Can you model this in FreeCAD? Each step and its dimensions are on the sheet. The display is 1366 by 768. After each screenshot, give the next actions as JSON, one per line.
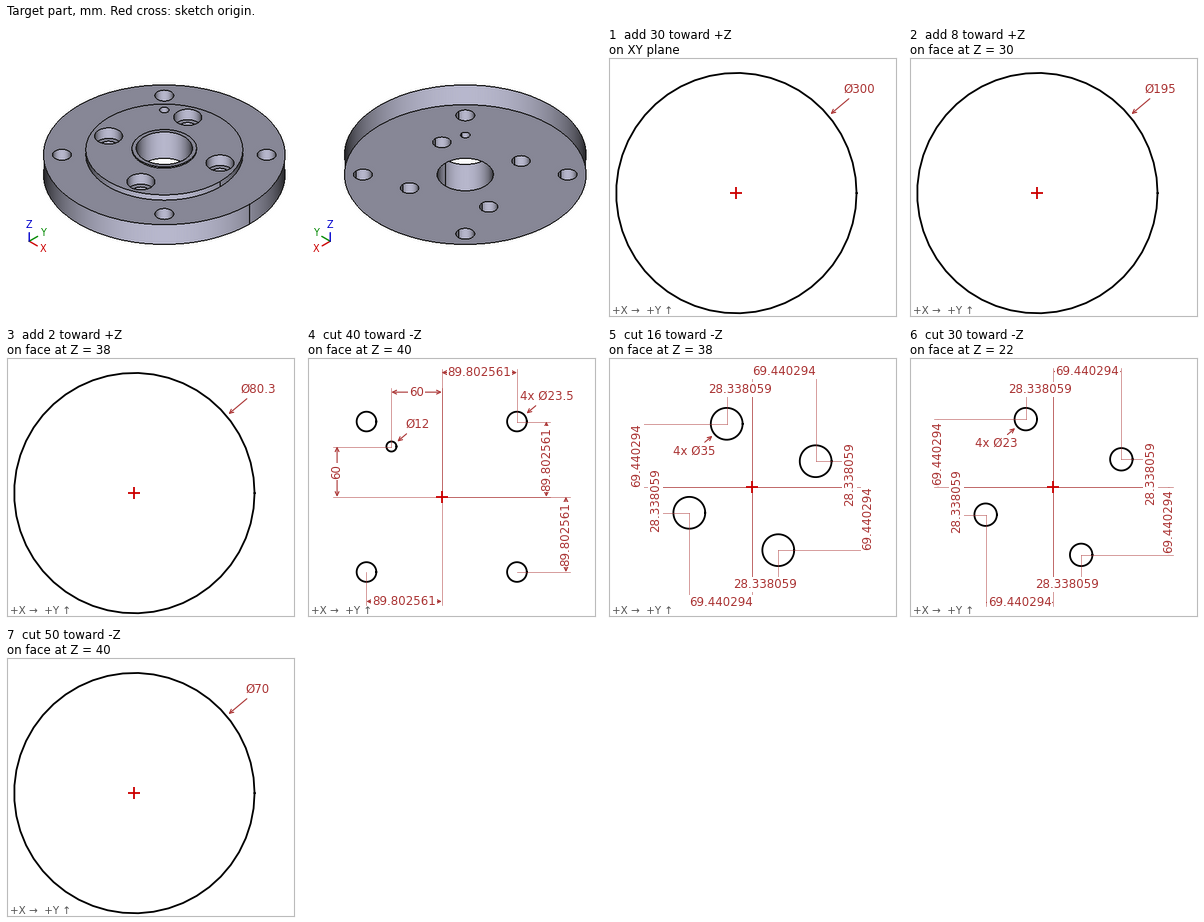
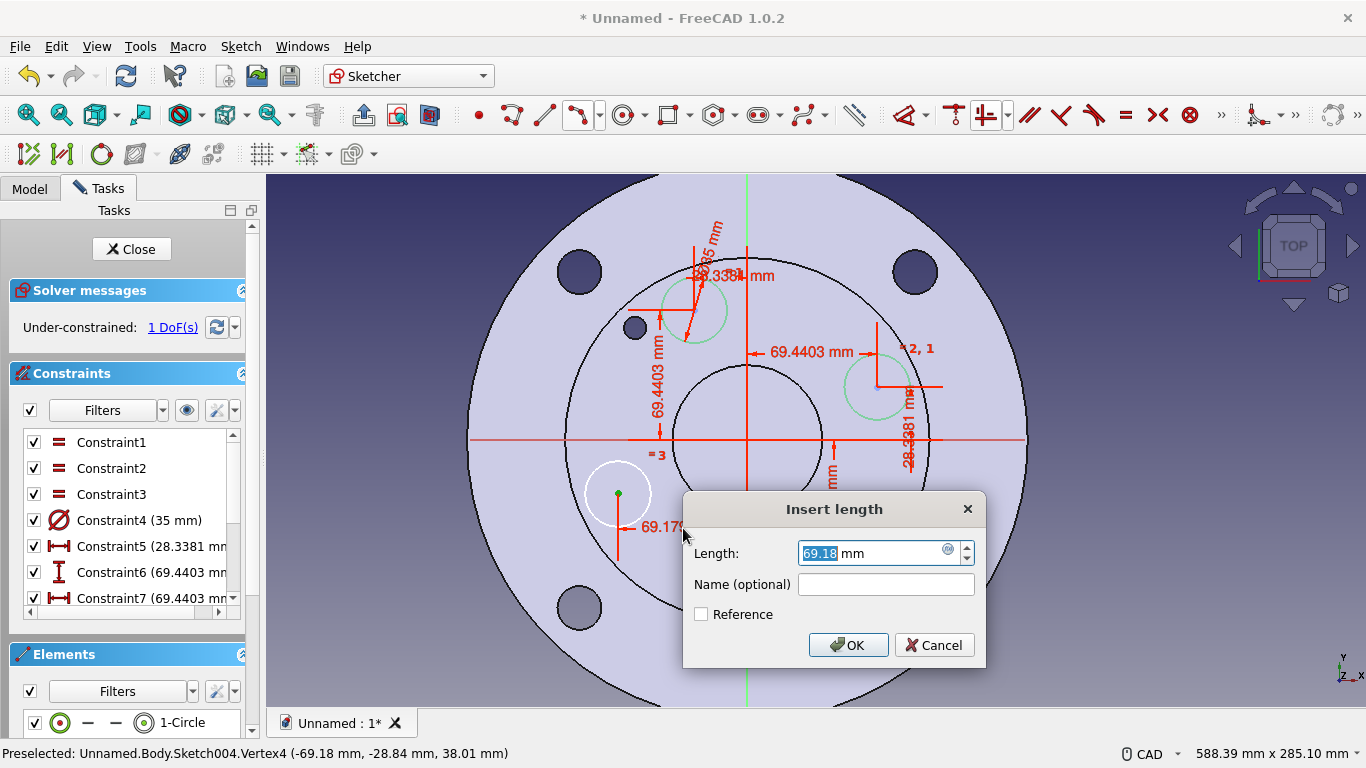
{"action": "type", "text": "69.440294"}
{"action": "key", "text": "Return"}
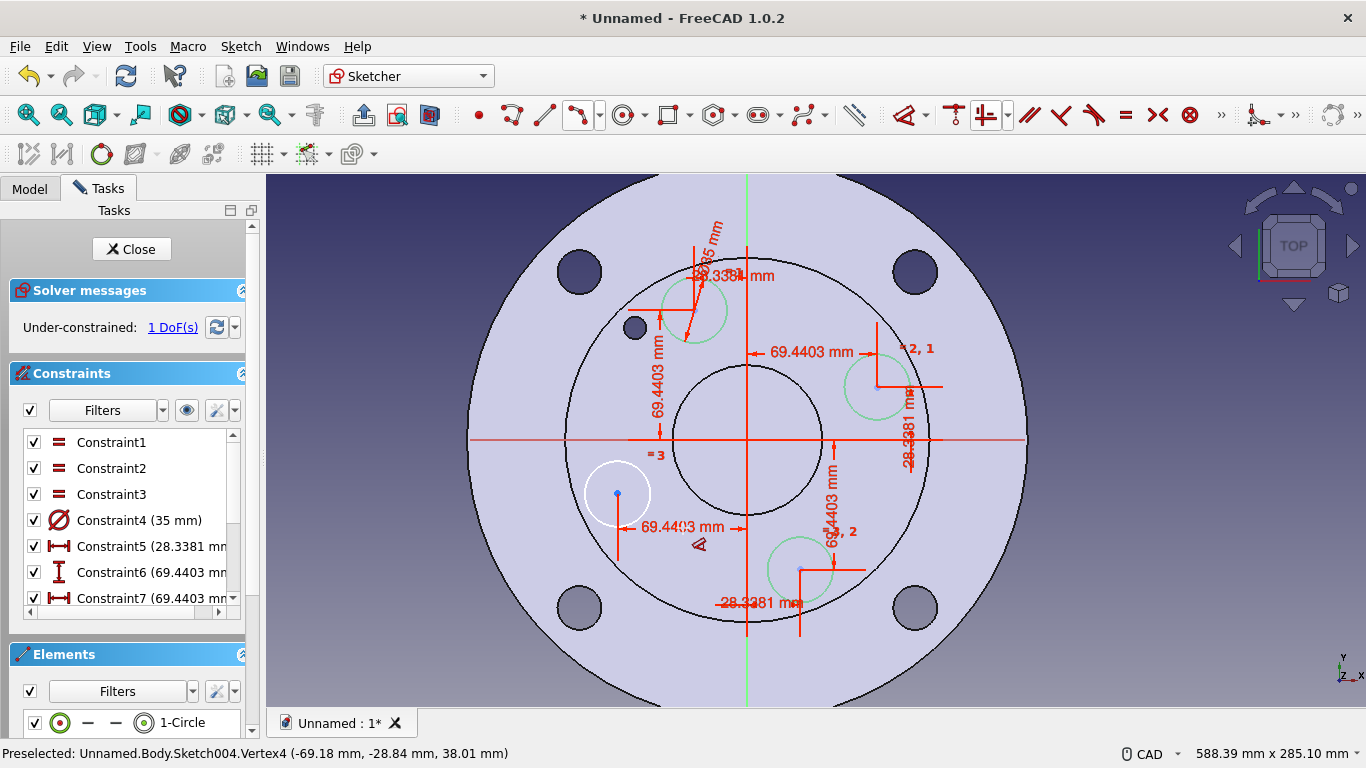
{"action": "left_click", "coordinate": [618, 494]}
{"action": "left_click", "coordinate": [584, 455]}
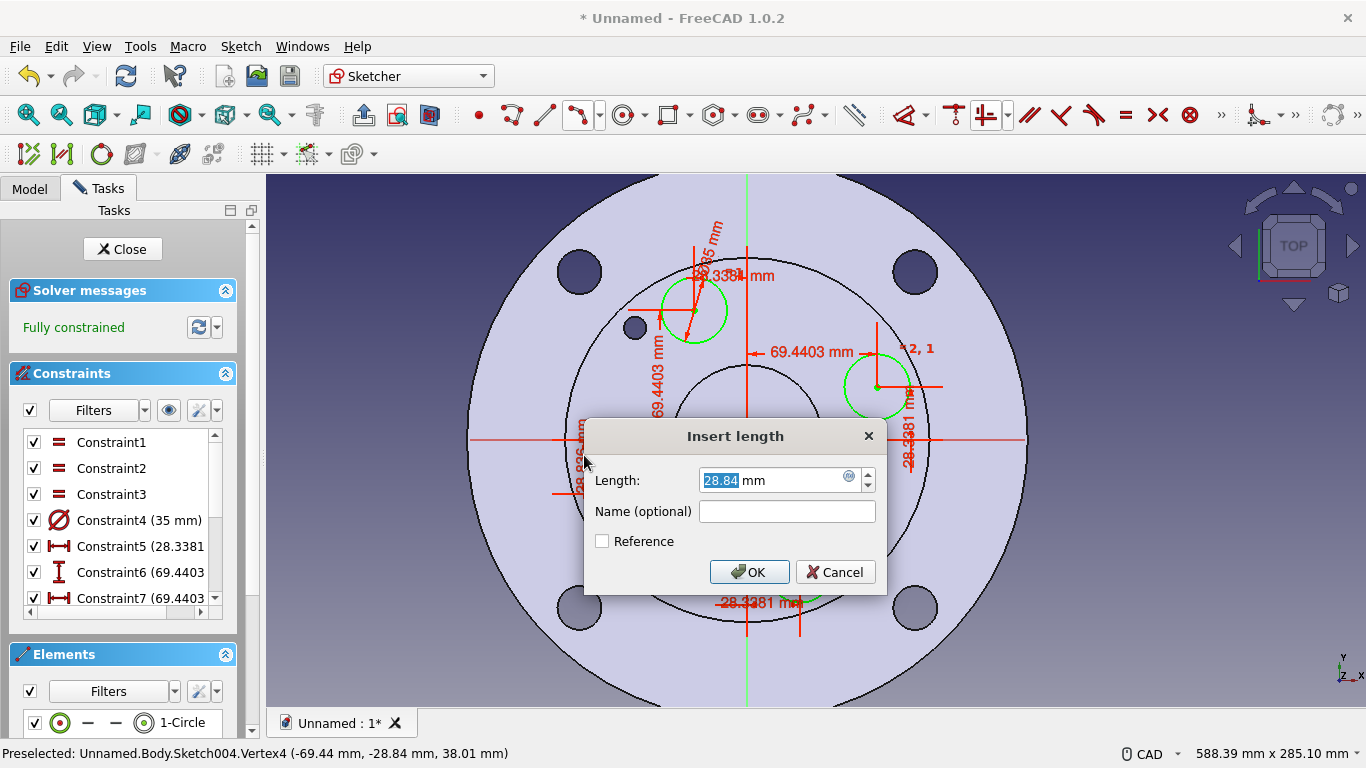
{"action": "type", "text": "28.338059"}
{"action": "key", "text": "Return"}
{"action": "key", "text": "Escape"}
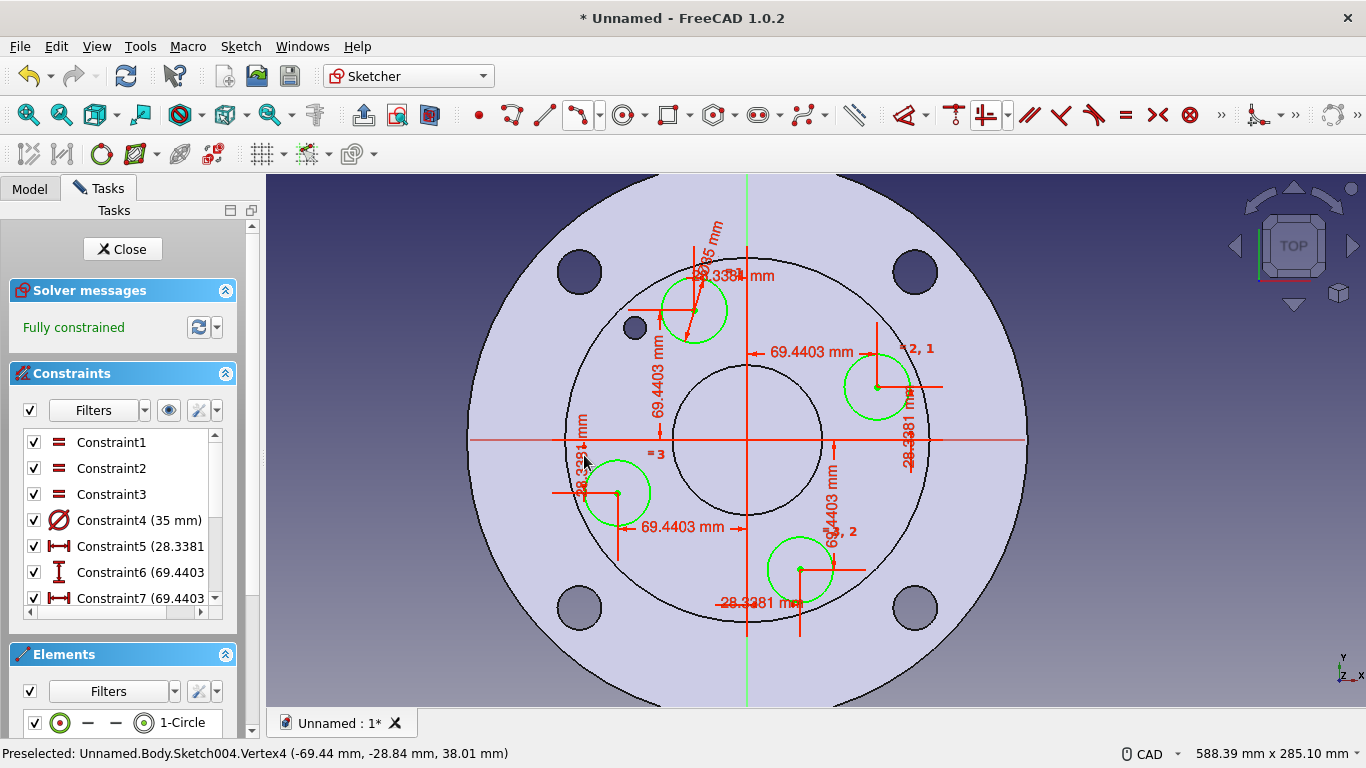
{"action": "left_click", "coordinate": [123, 249]}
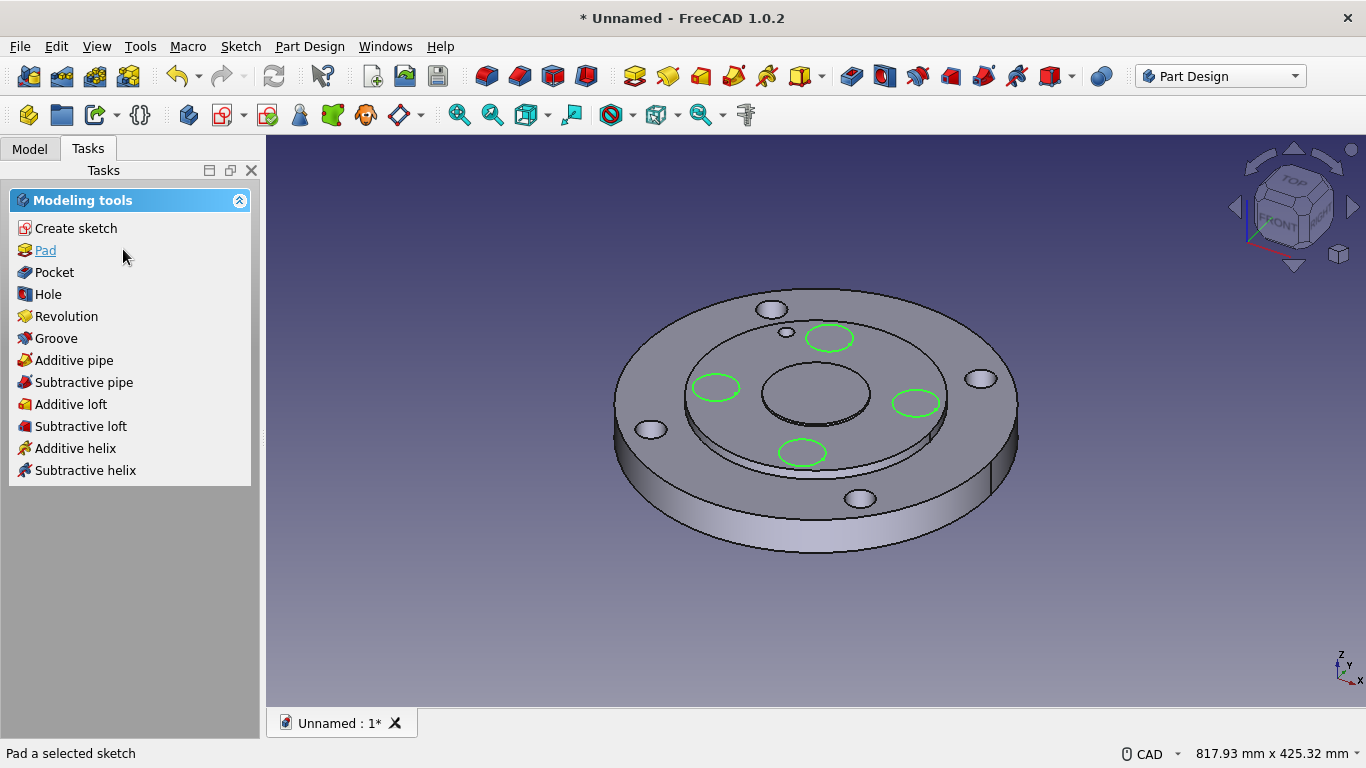
{"action": "left_click", "coordinate": [852, 76]}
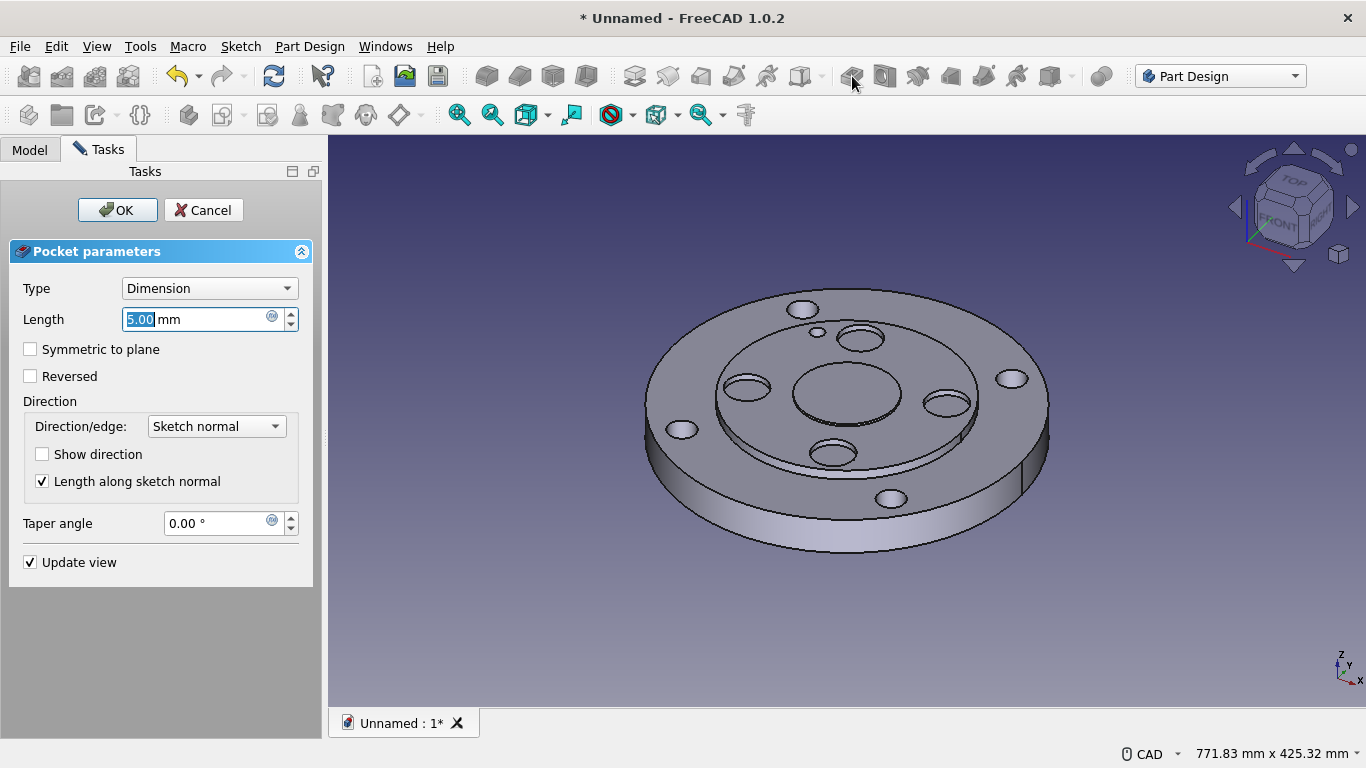
{"action": "type", "text": "16"}
{"action": "key", "text": "Tab"}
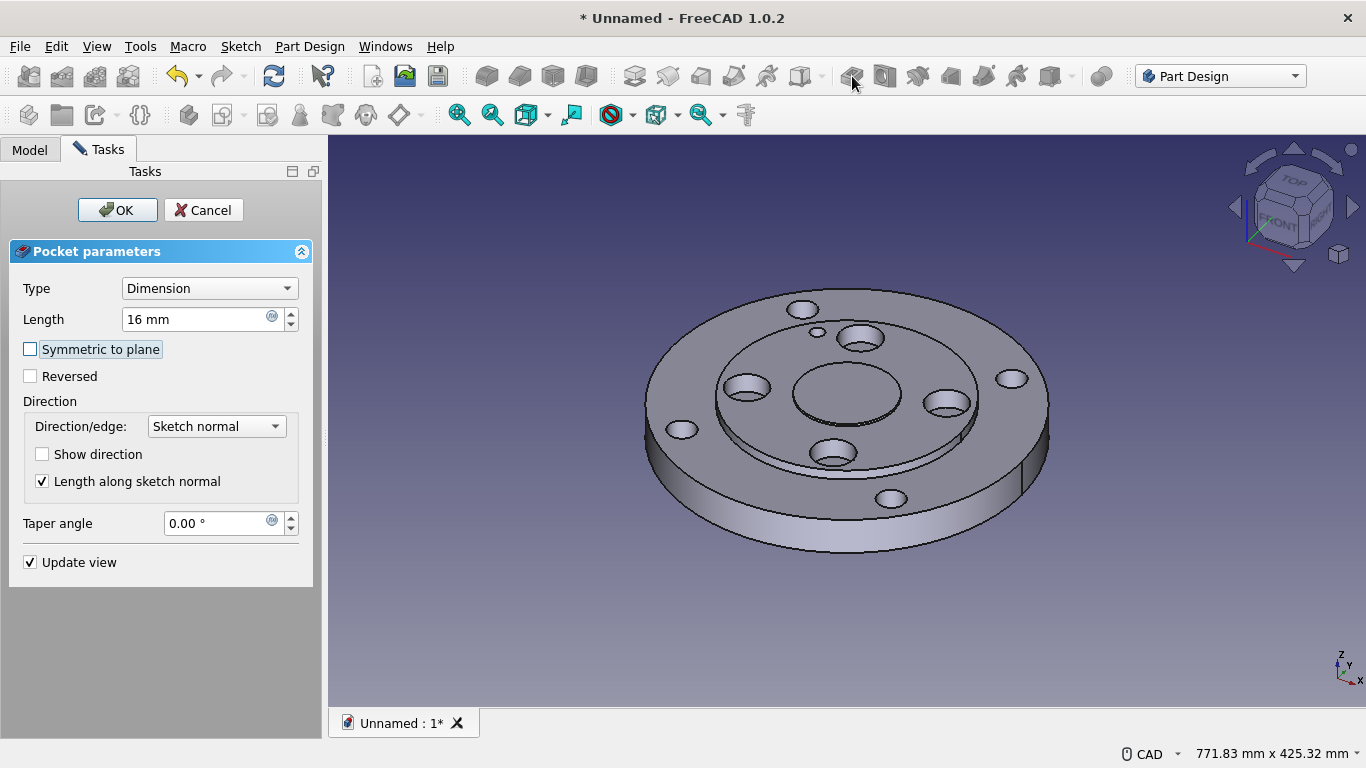
{"action": "left_click", "coordinate": [118, 210]}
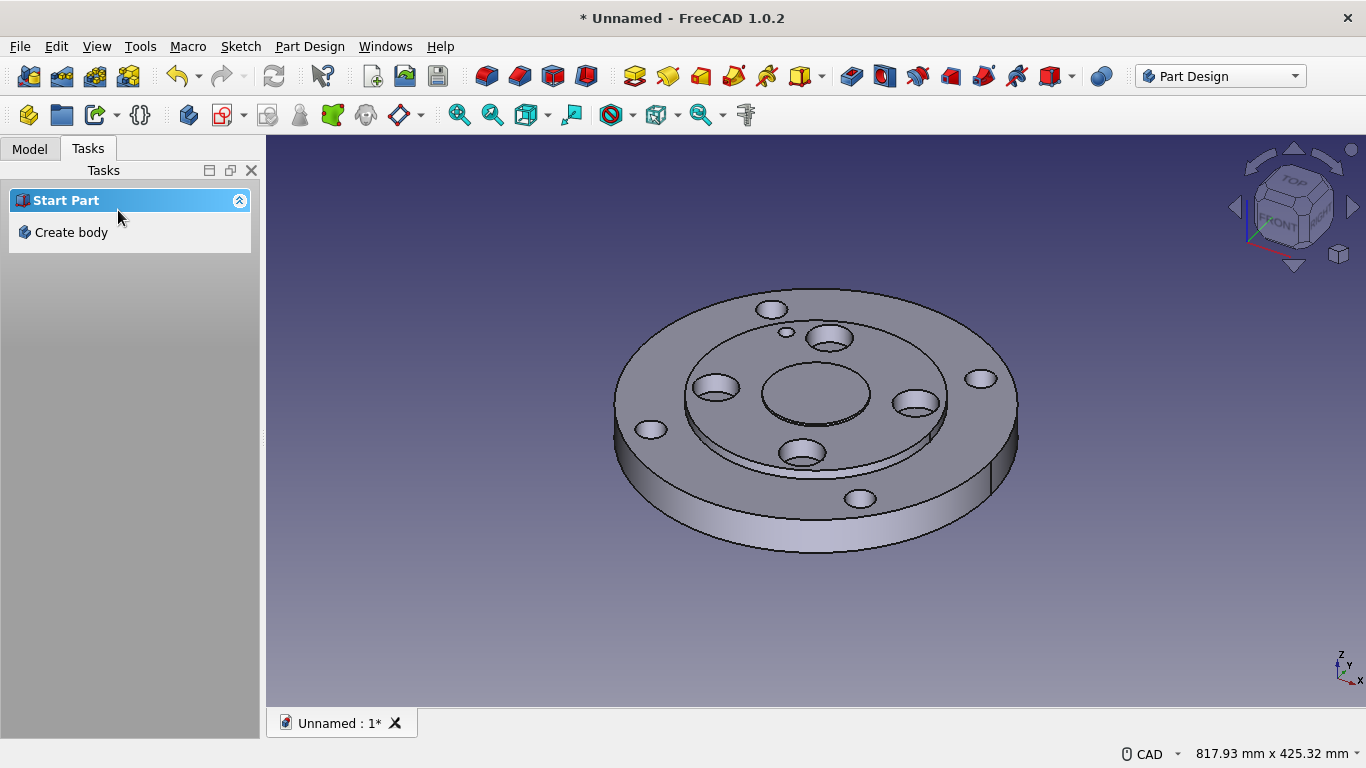
{"action": "key", "text": "0"}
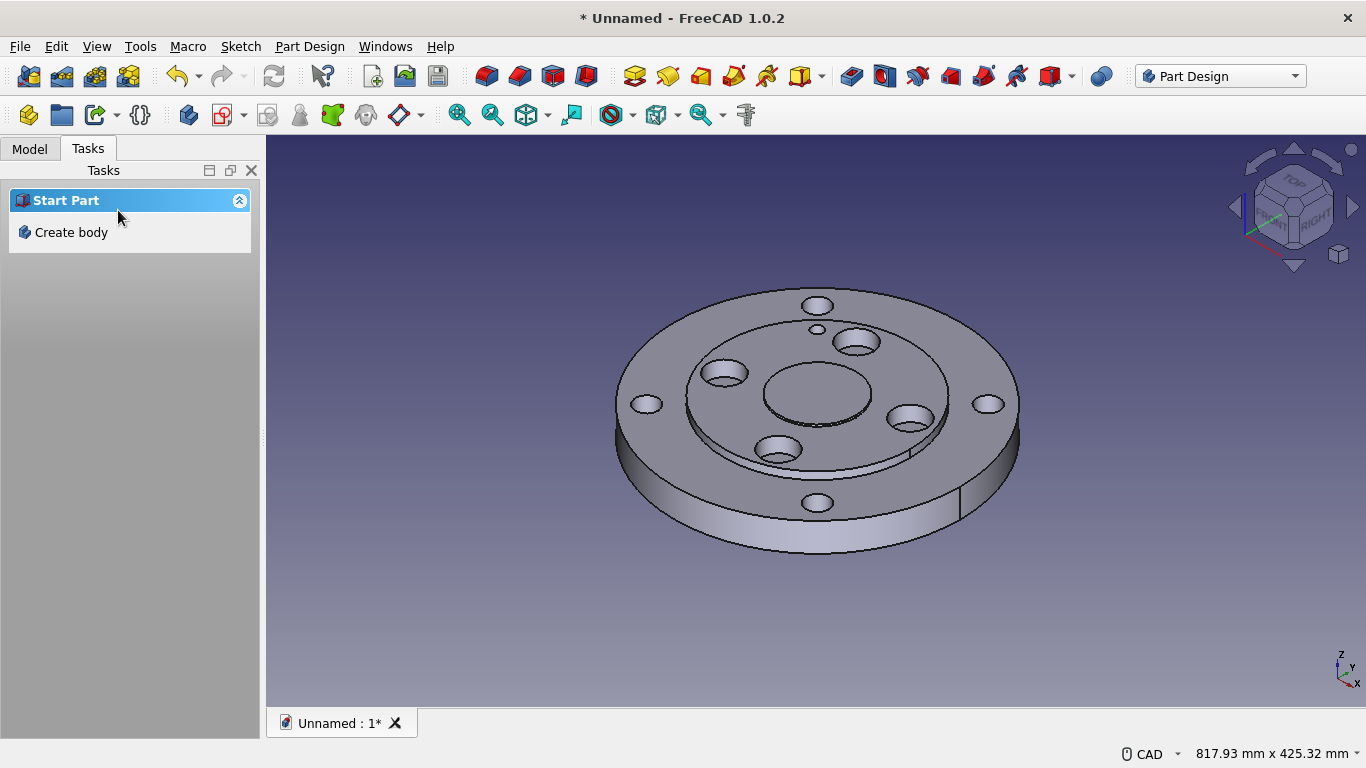
{"action": "key", "text": "2"}